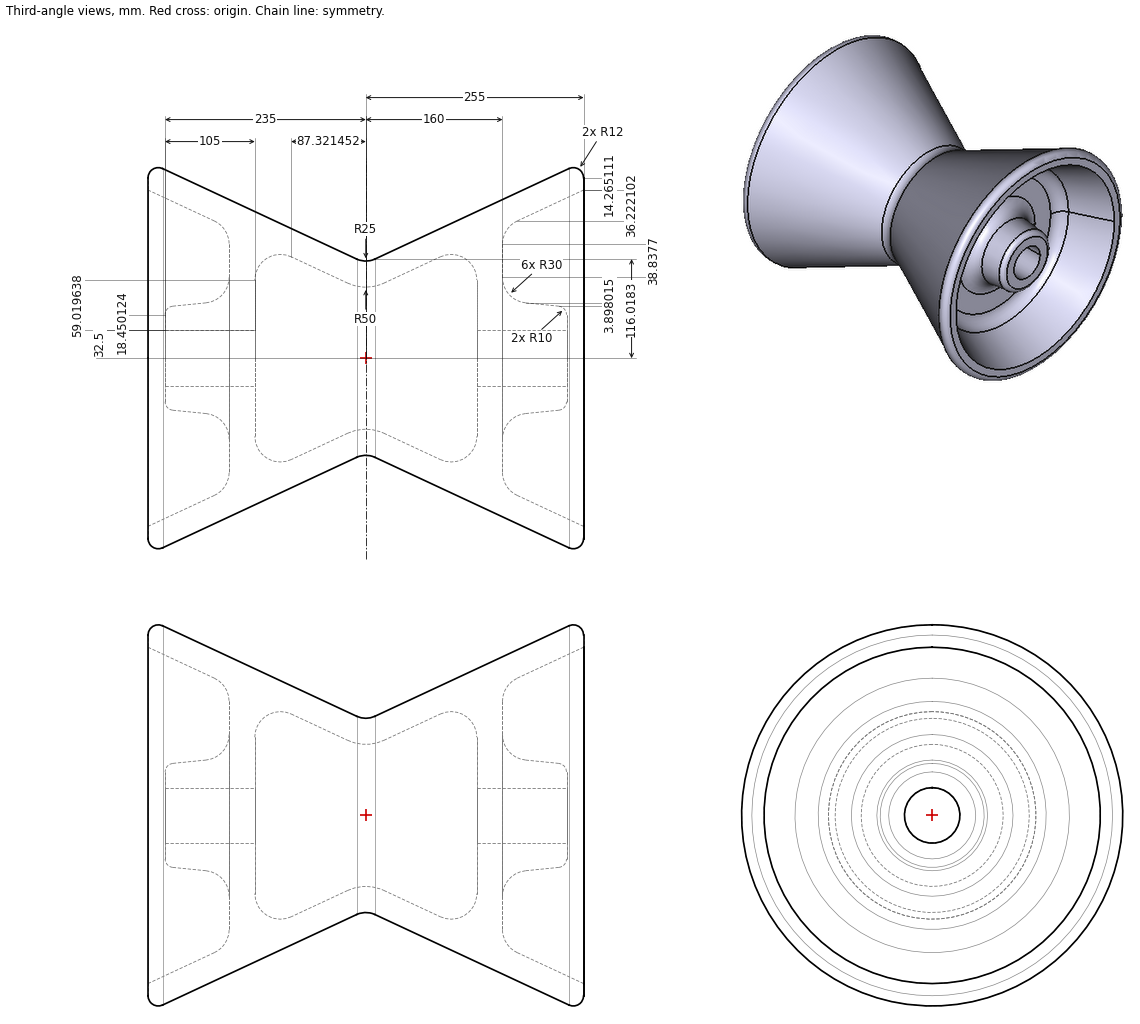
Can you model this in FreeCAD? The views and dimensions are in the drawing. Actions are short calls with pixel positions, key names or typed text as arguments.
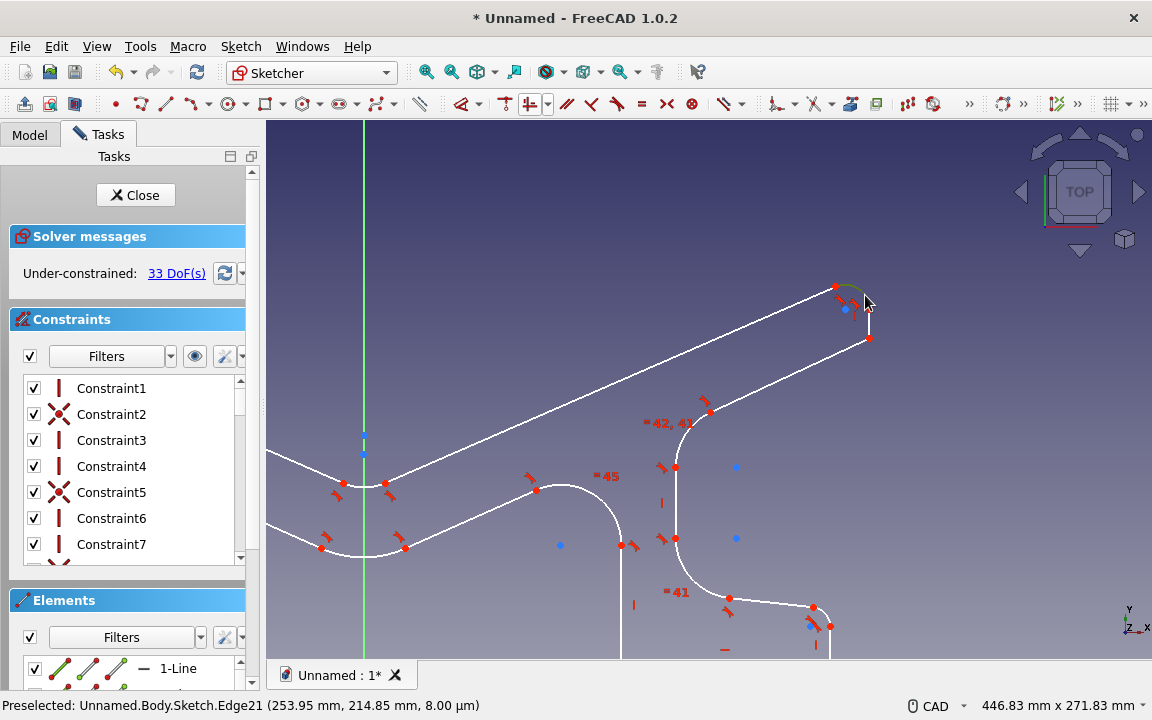
scroll(866, 295, down, 4)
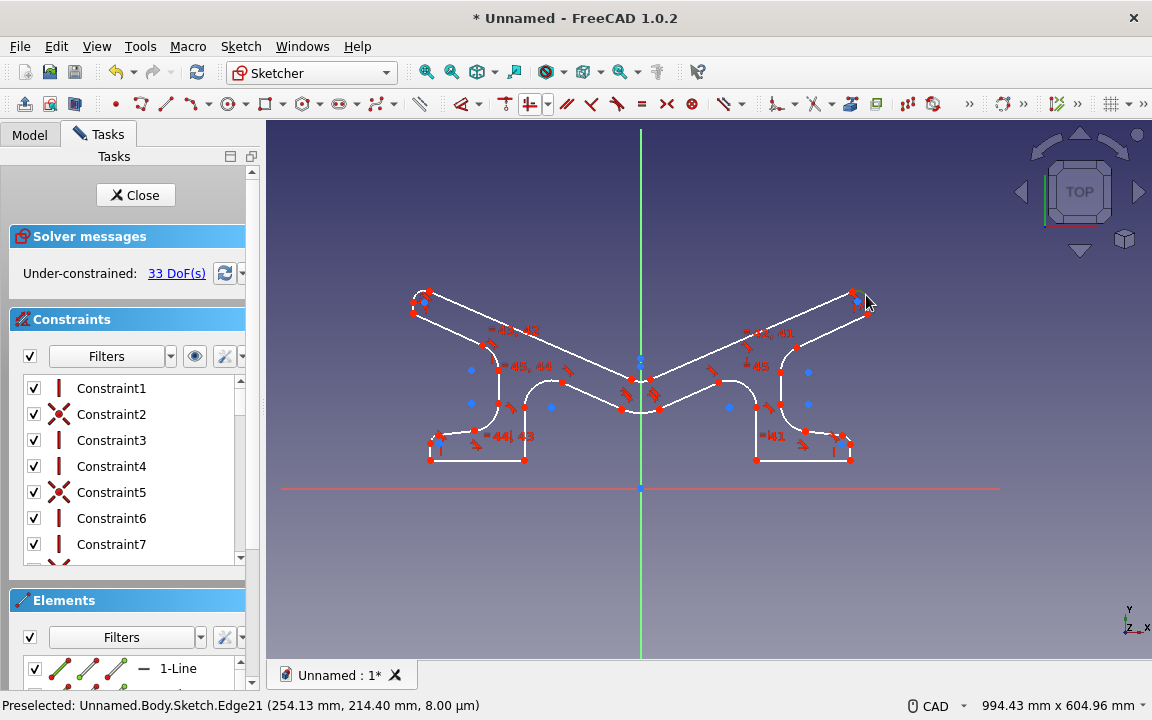
scroll(423, 291, up, 4)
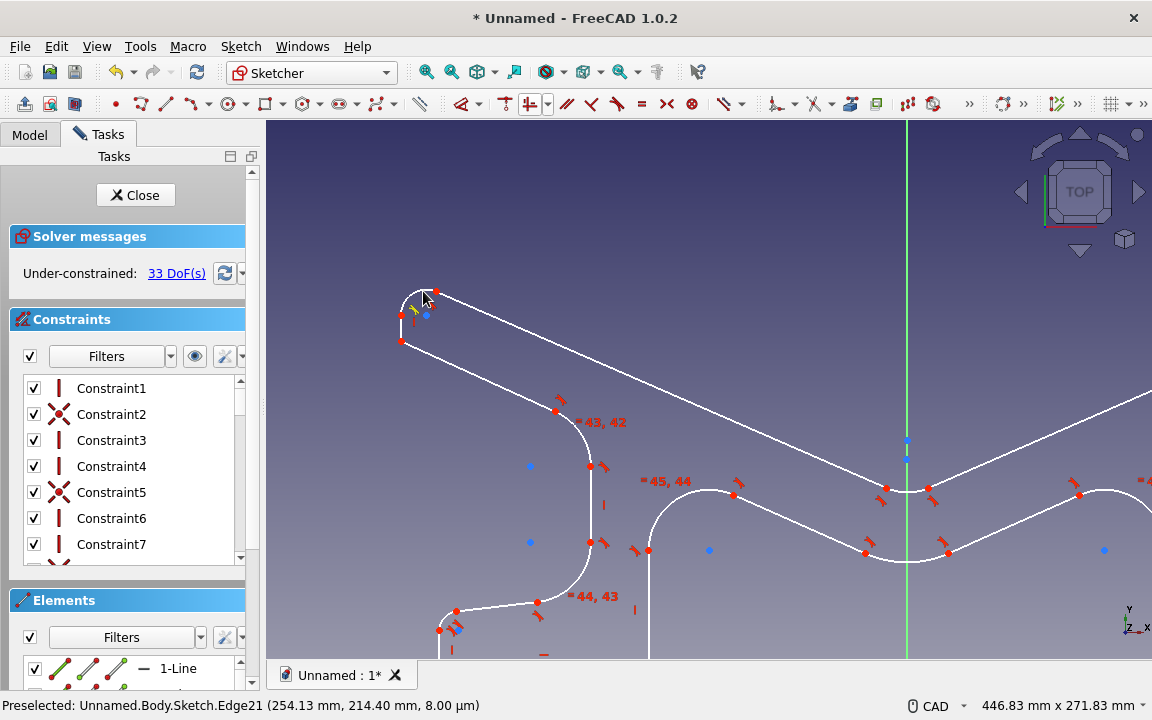
click(422, 290)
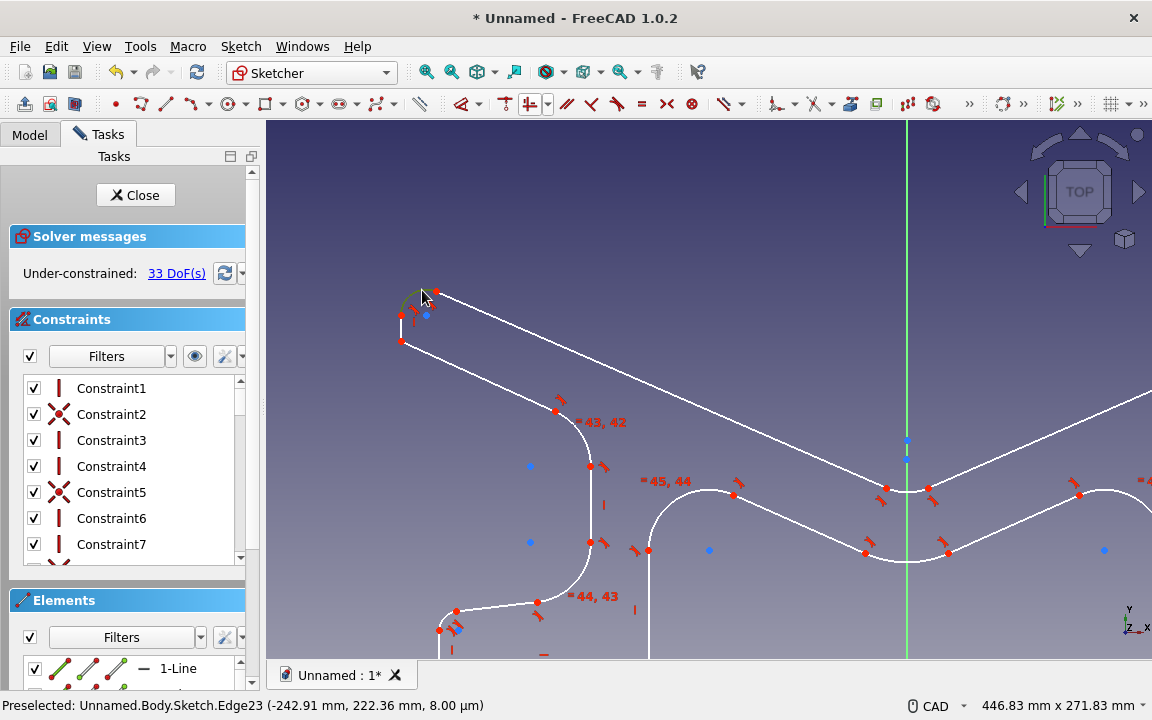
click(642, 104)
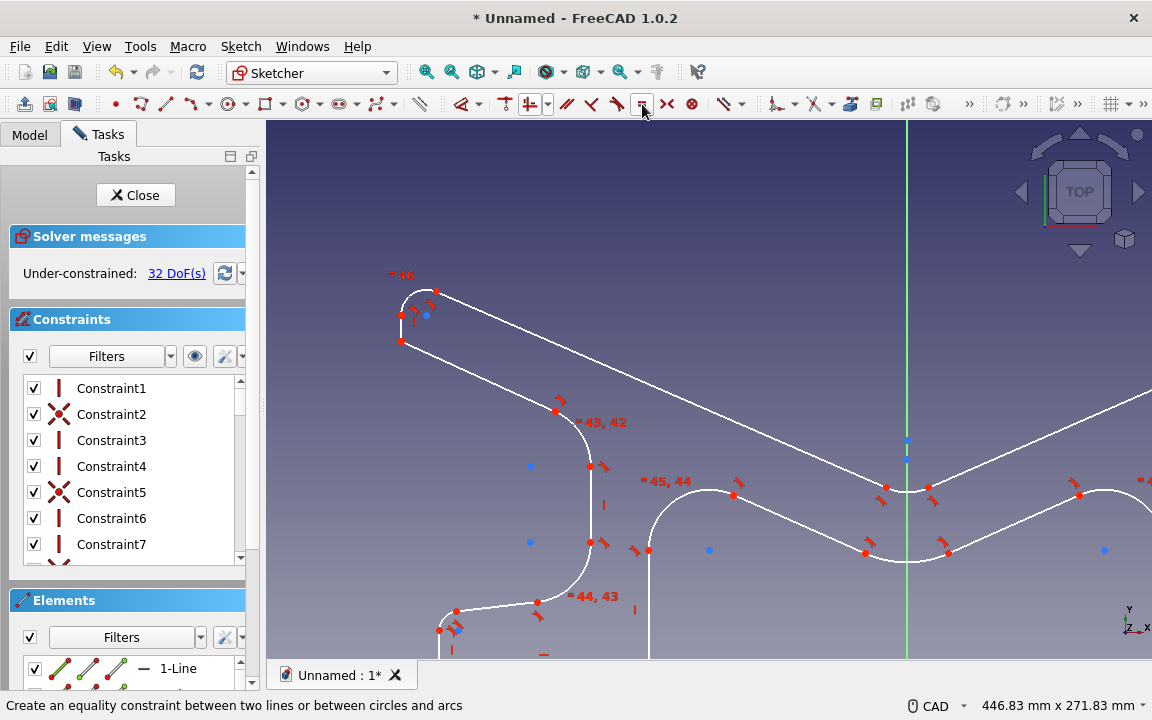
click(444, 618)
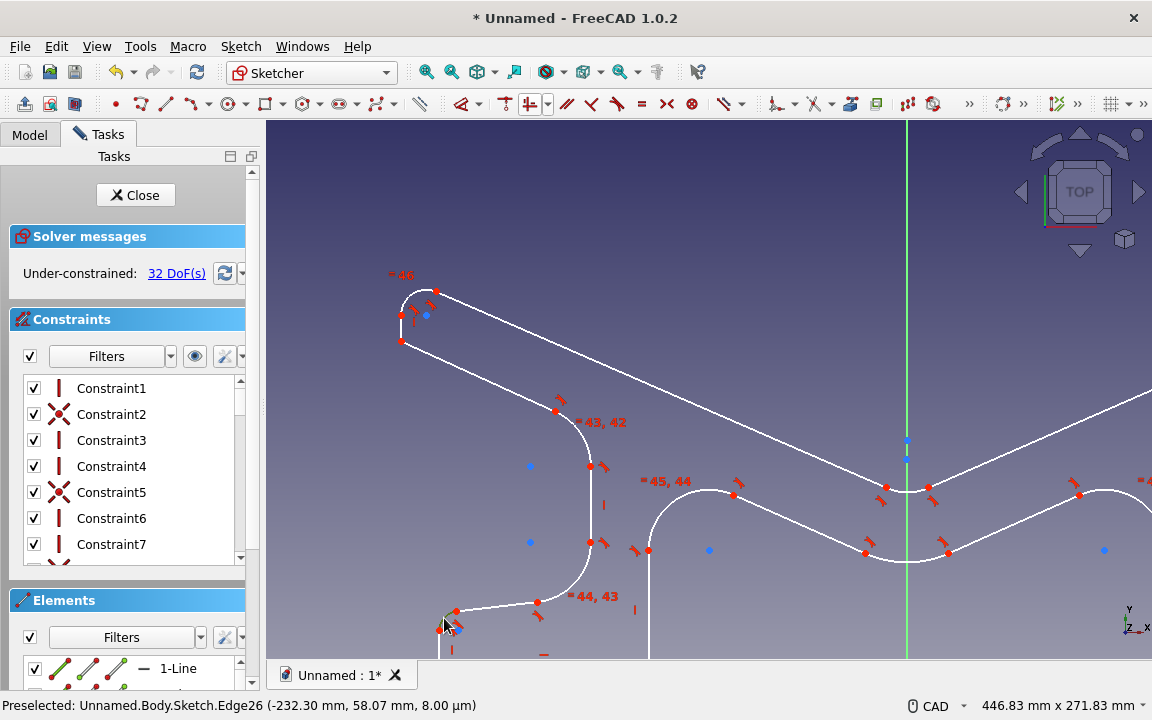
scroll(423, 291, down, 4)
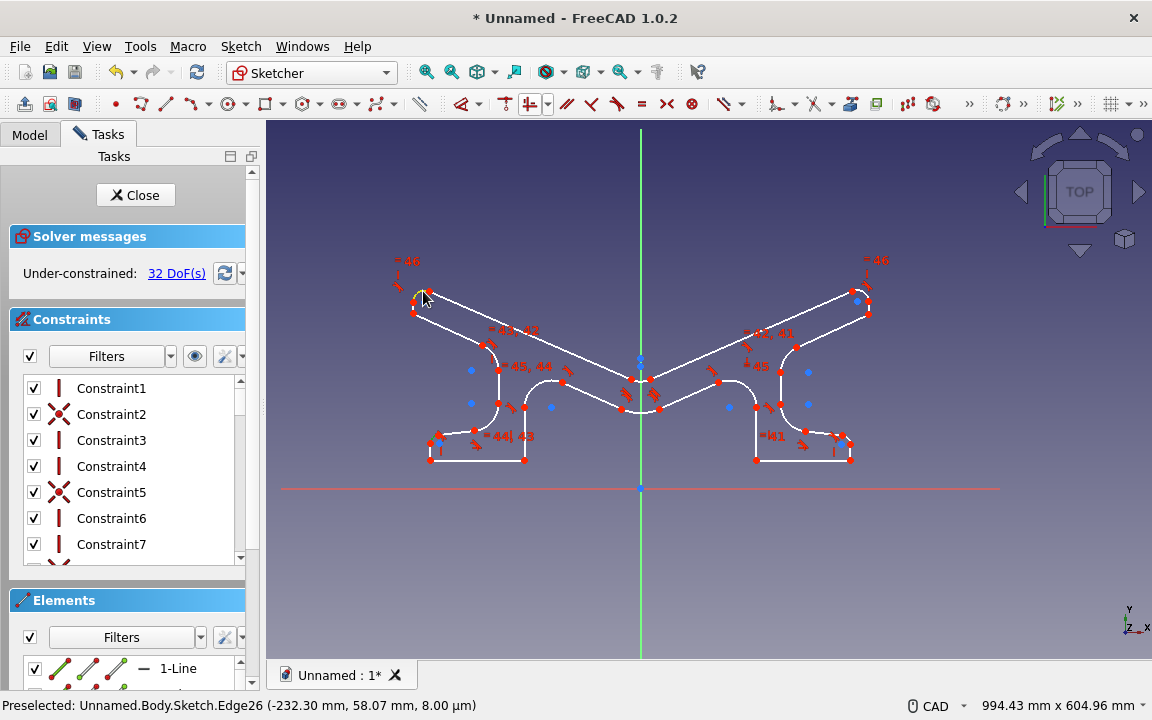
scroll(848, 438, up, 5)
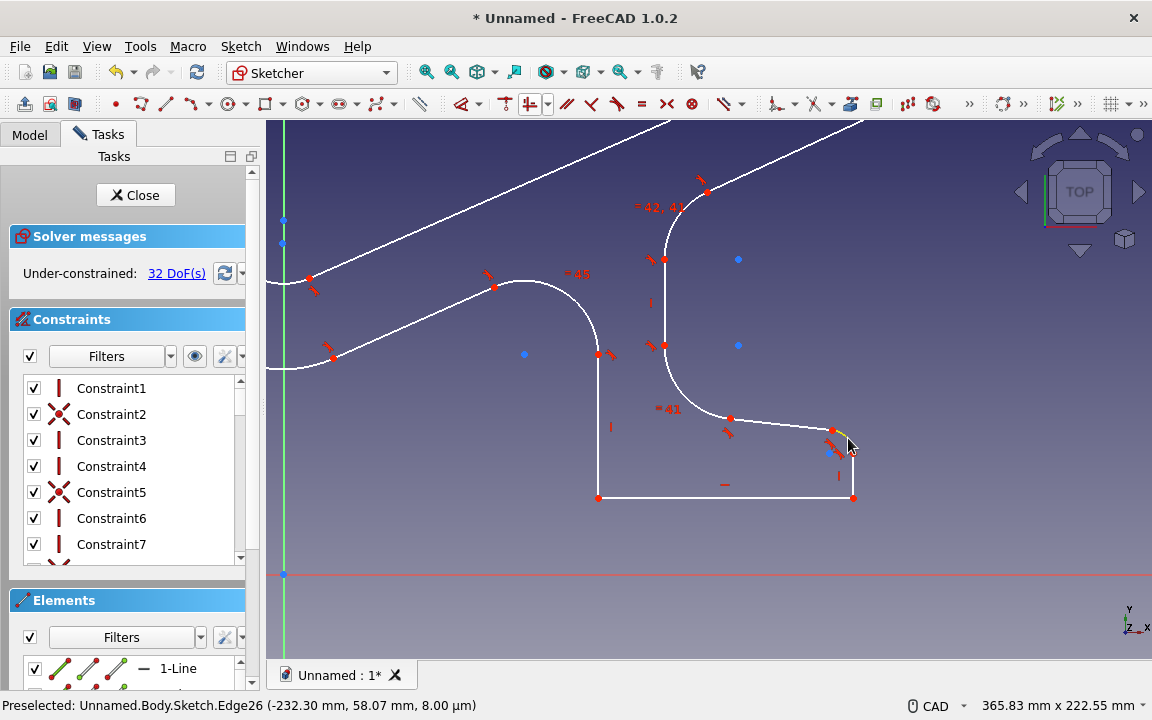
click(847, 438)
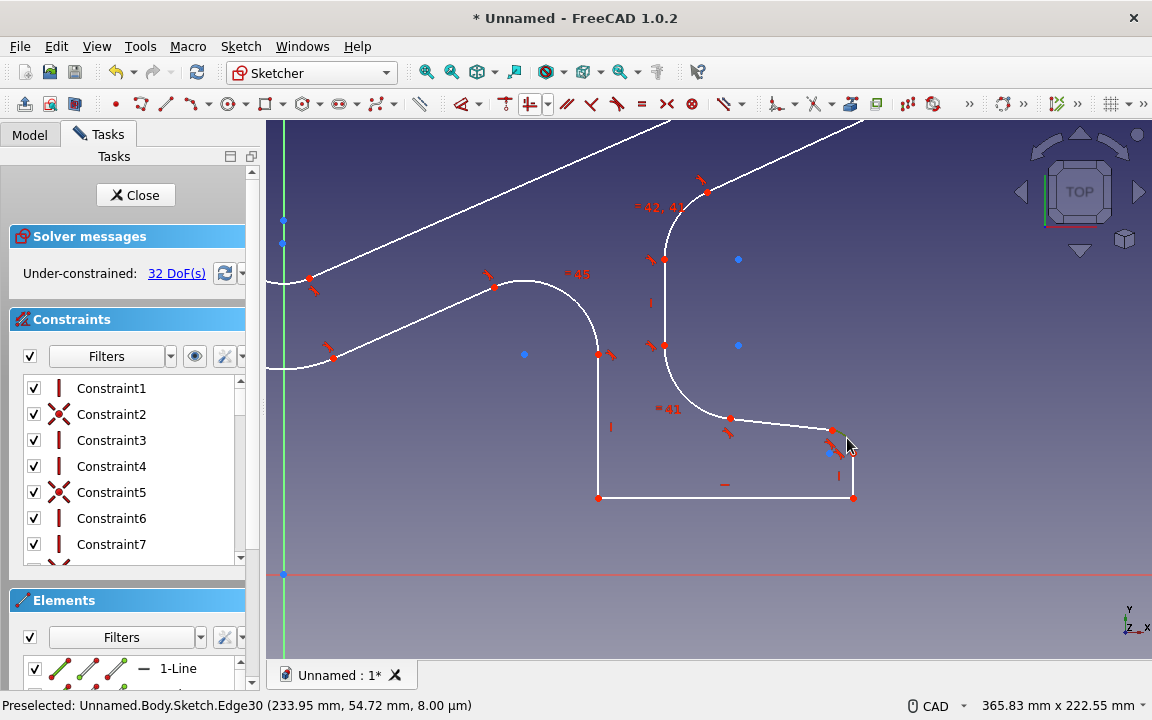
click(642, 104)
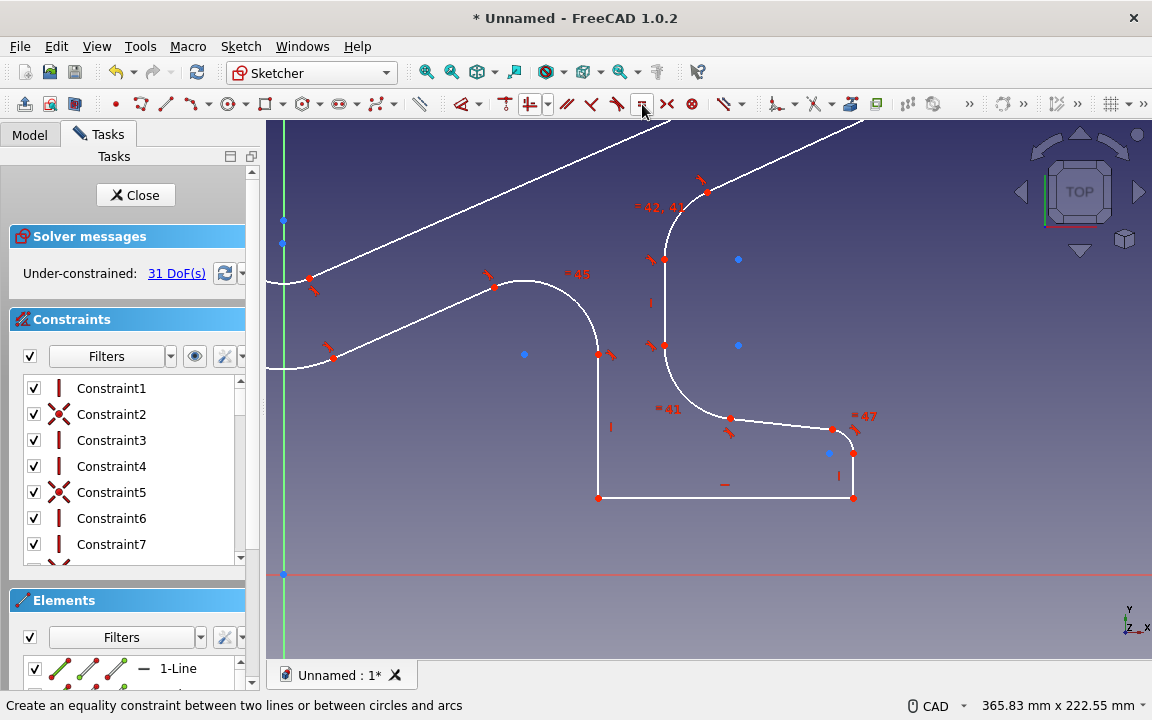
scroll(848, 438, down, 5)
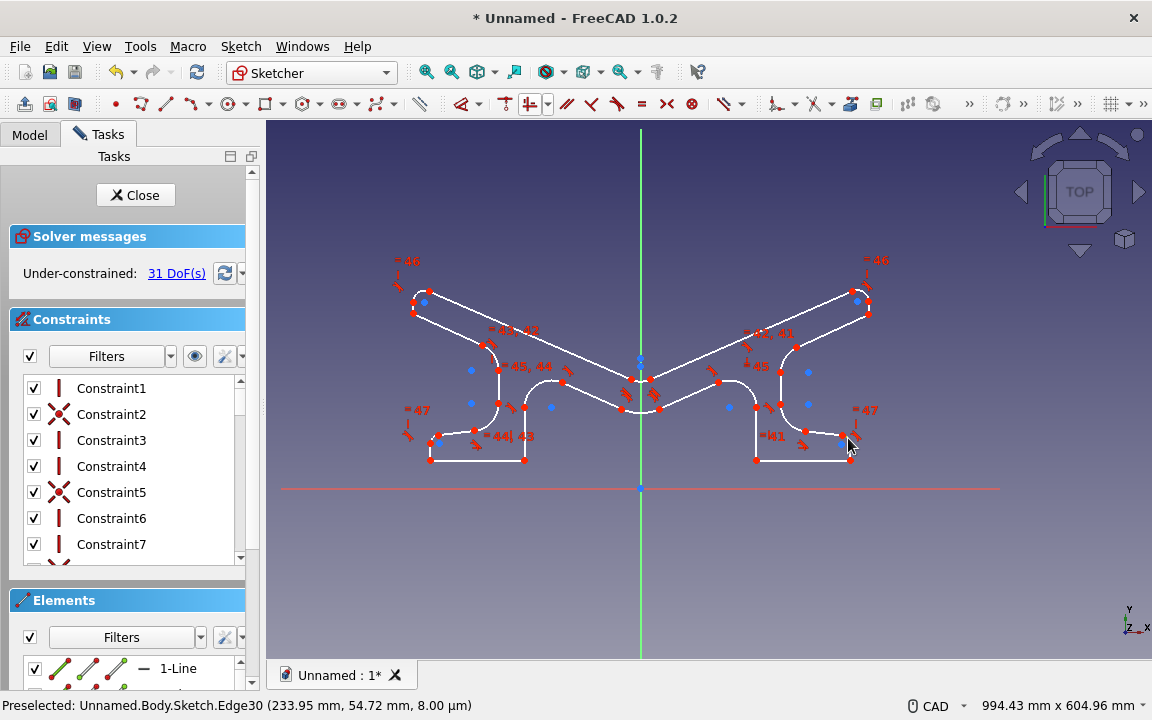
scroll(641, 358, up, 2)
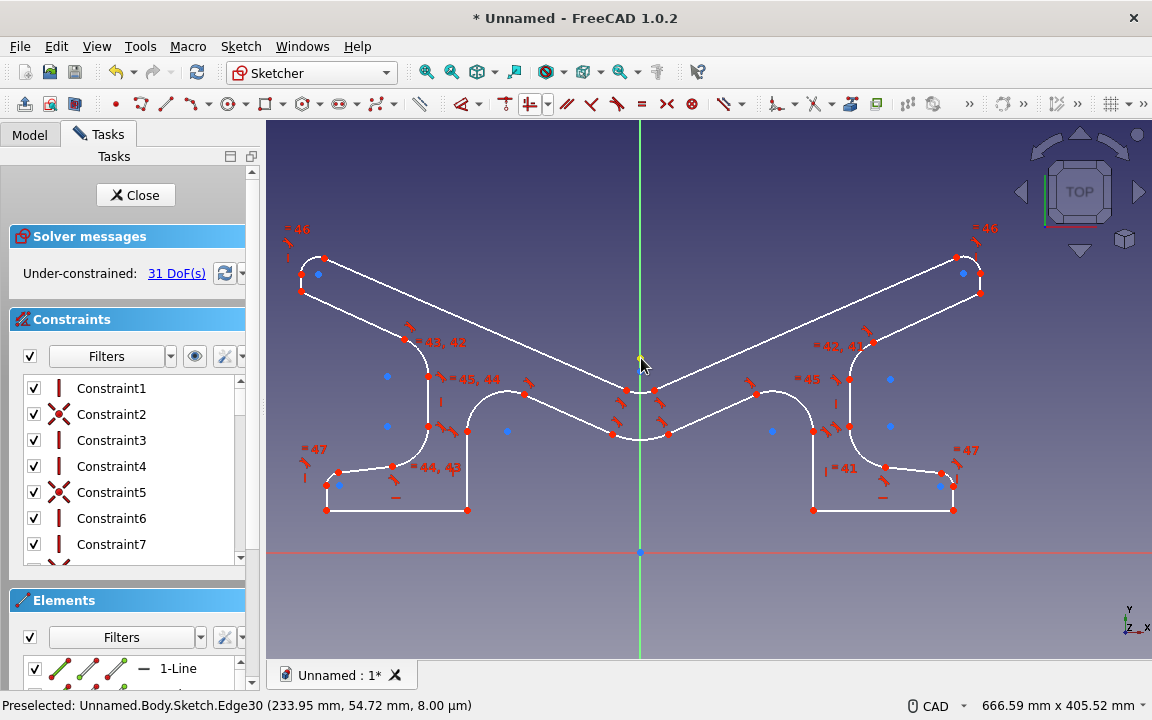
click(641, 358)